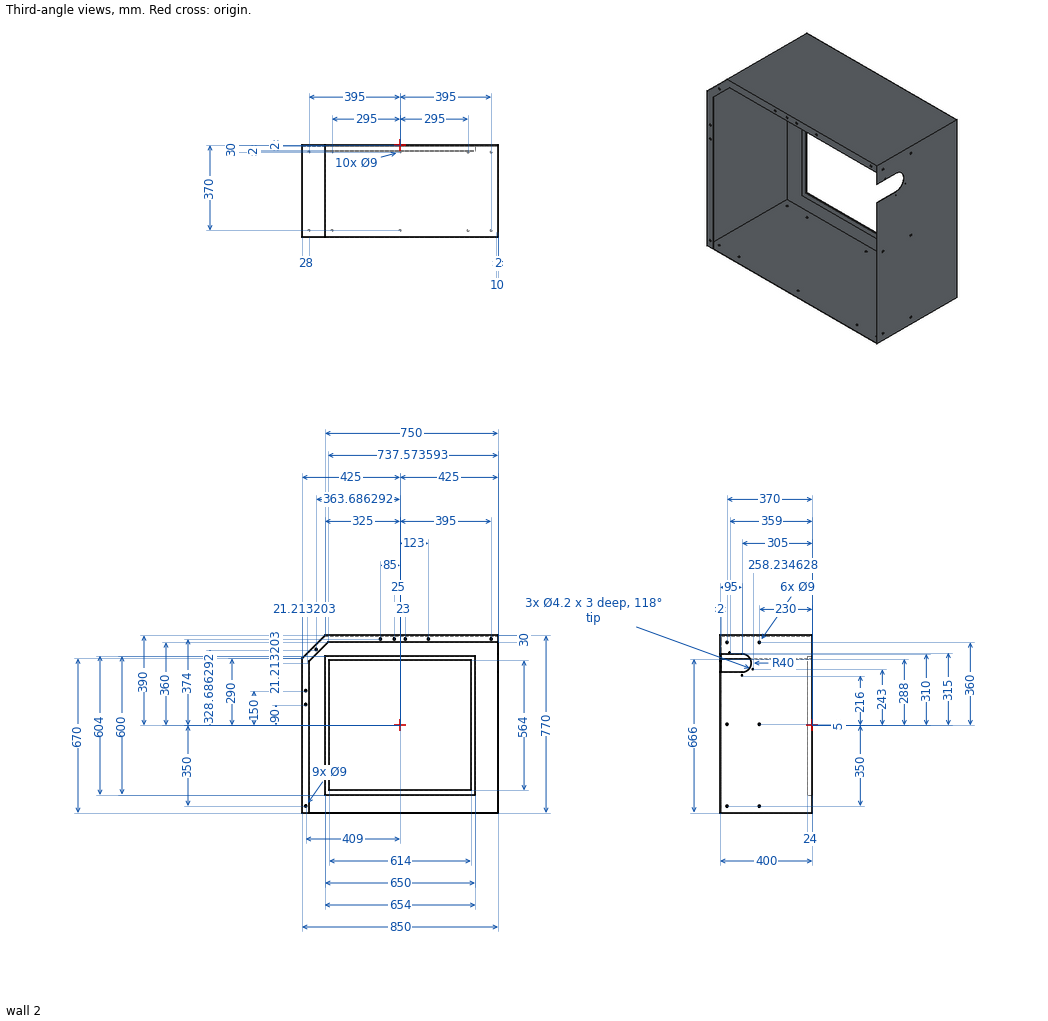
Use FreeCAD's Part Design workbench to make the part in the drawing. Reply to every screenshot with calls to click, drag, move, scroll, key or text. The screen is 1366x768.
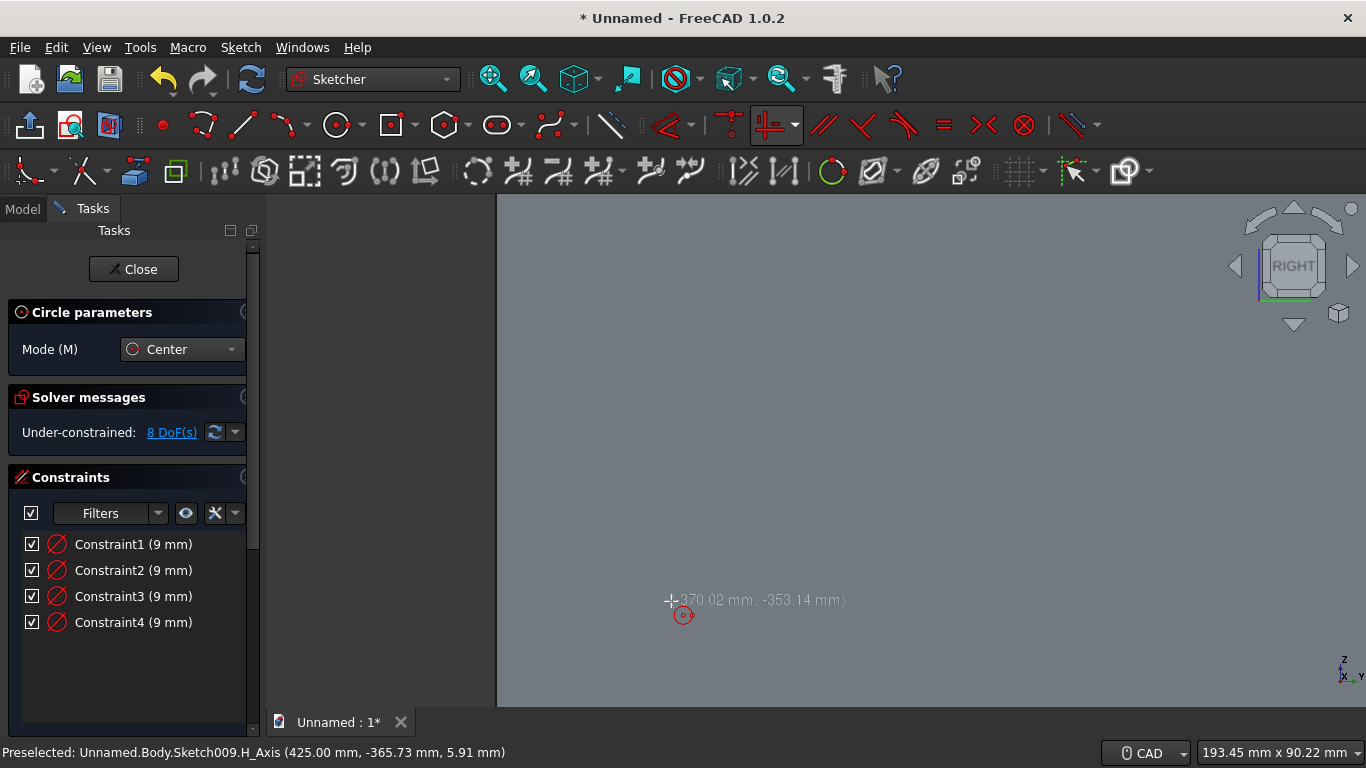
scroll(671, 602, down, 13)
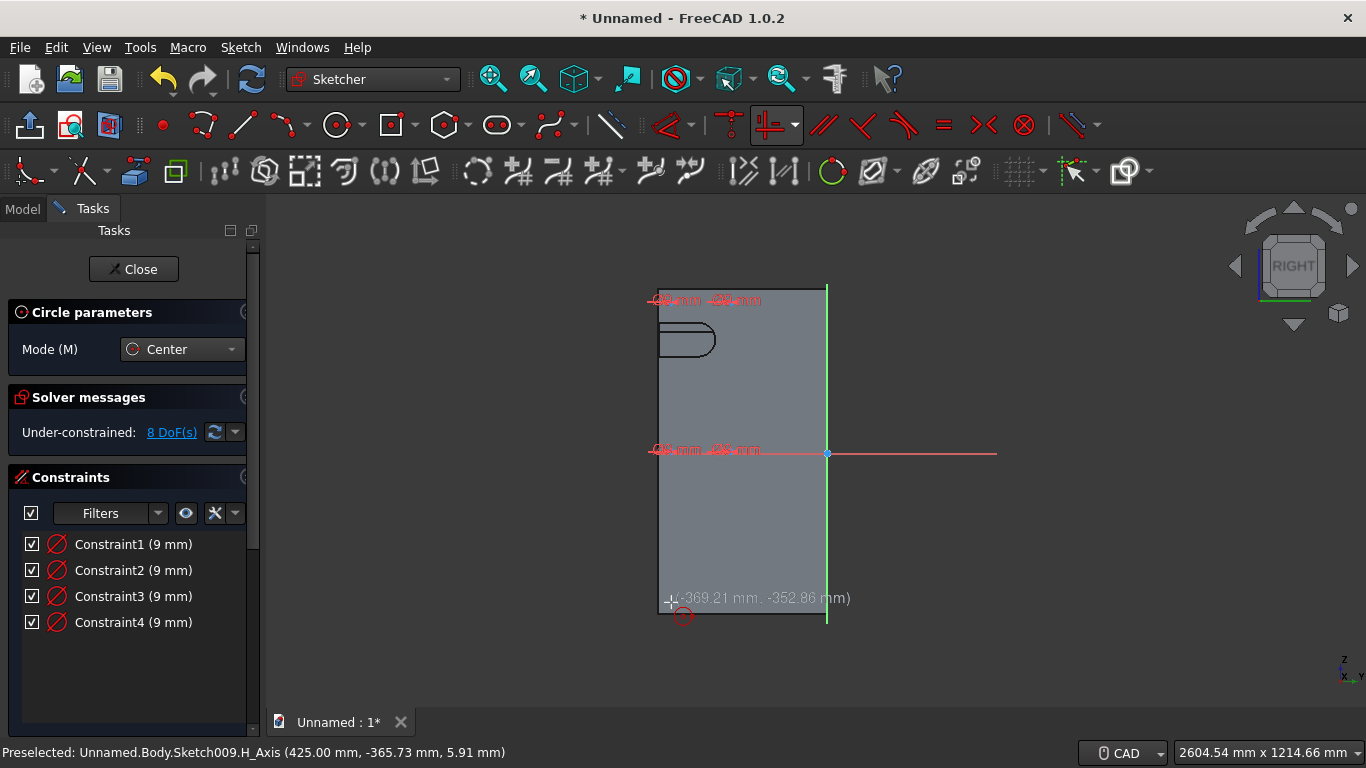
click(671, 602)
move(672, 600)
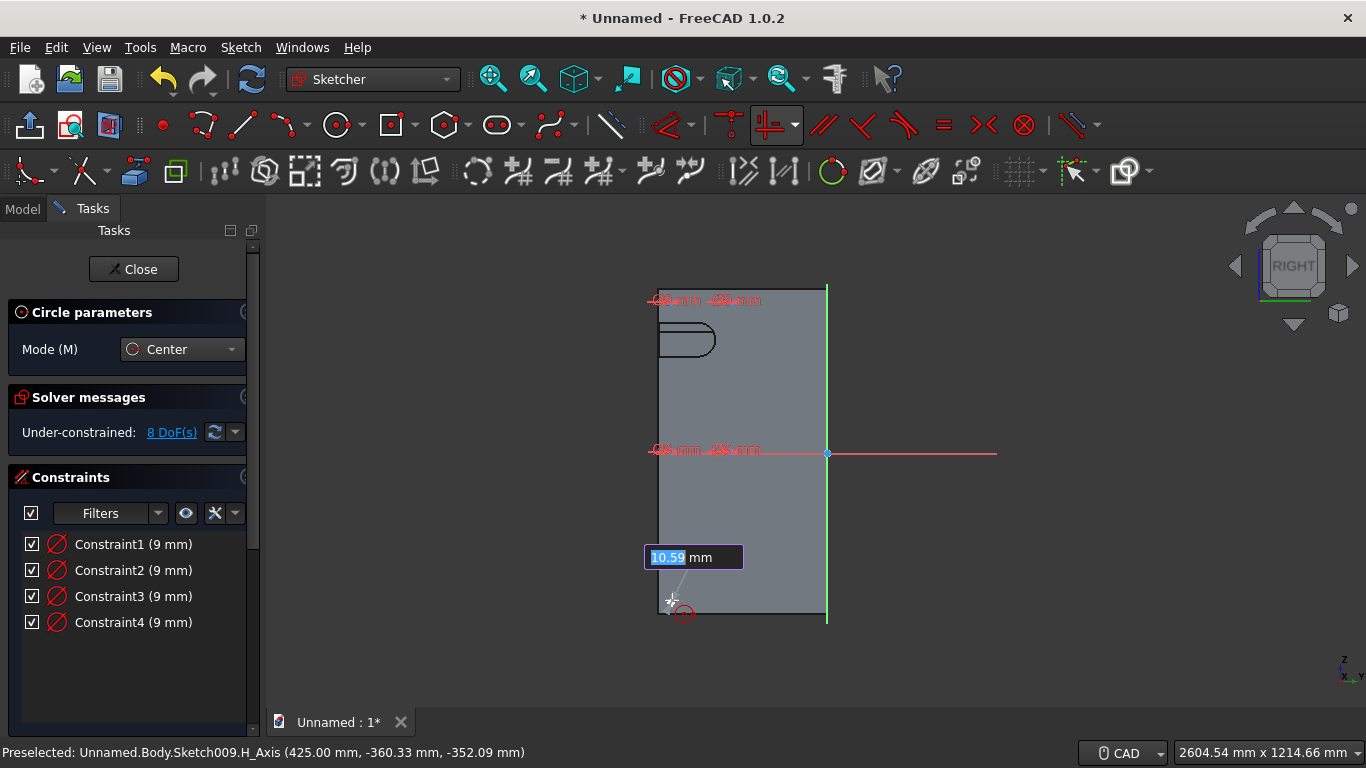
text(9)
key(Return)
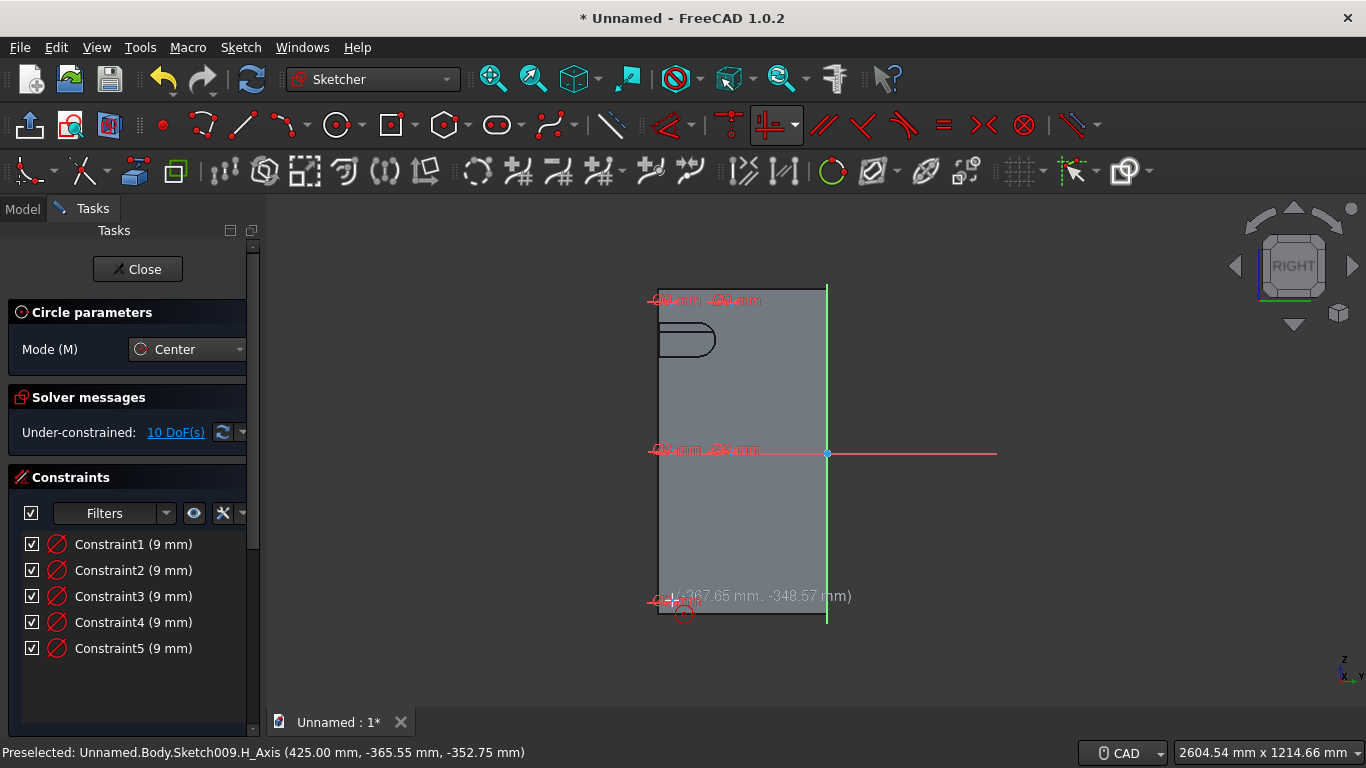
scroll(730, 602, up, 13)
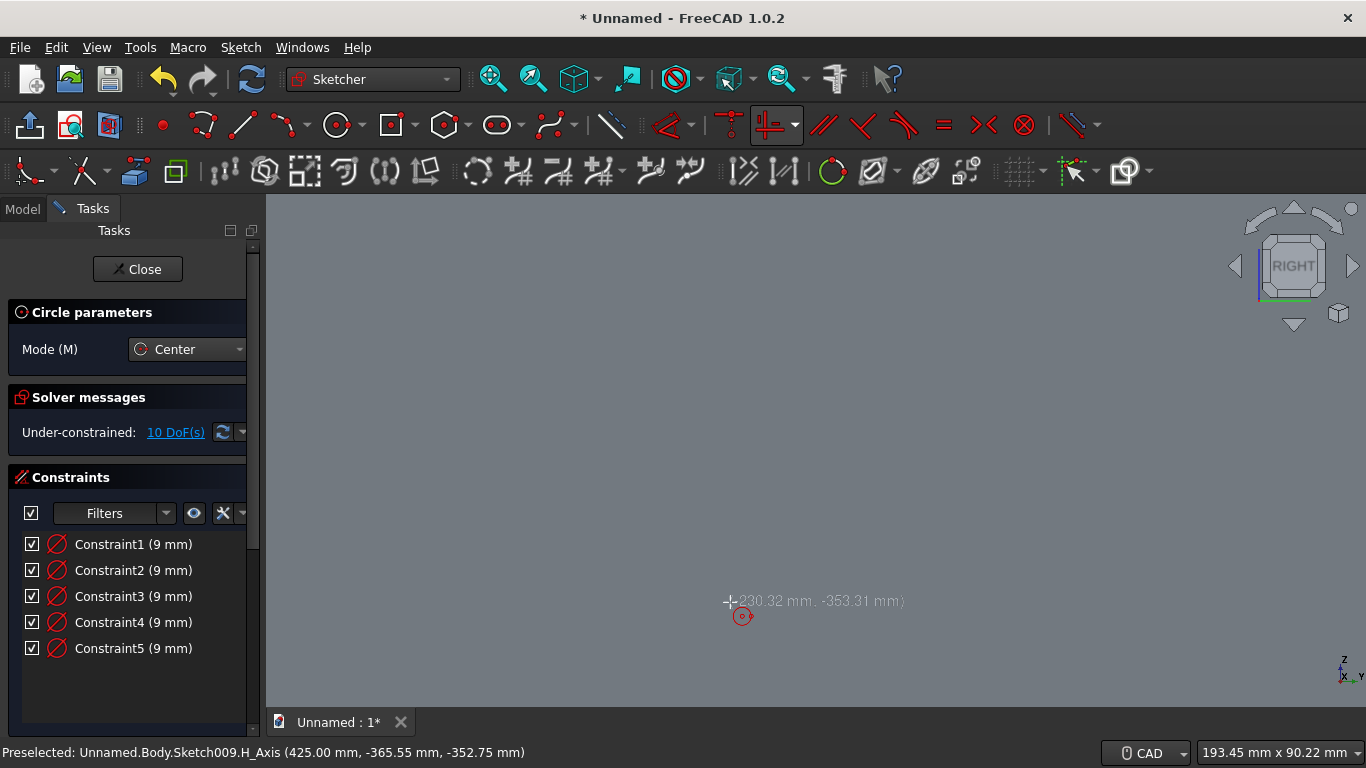
scroll(730, 602, down, 13)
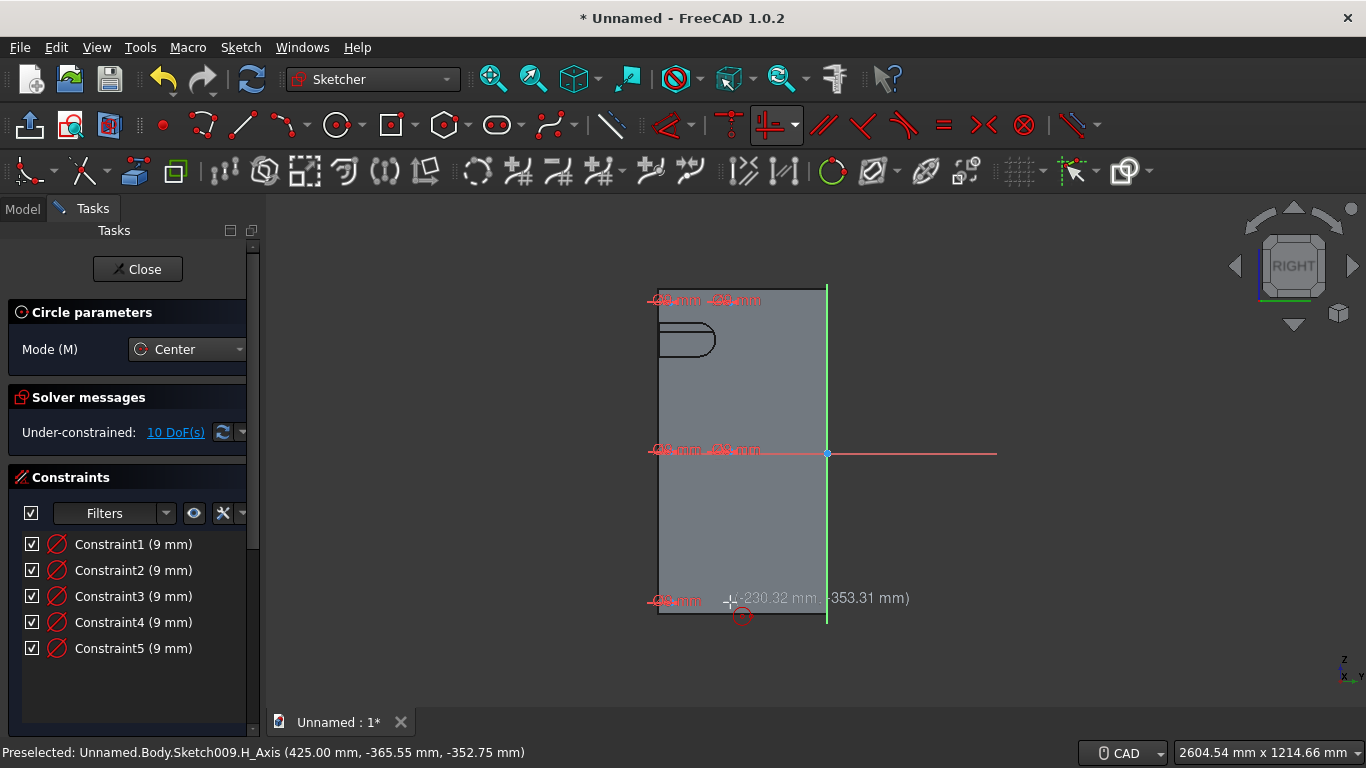
click(730, 602)
move(731, 600)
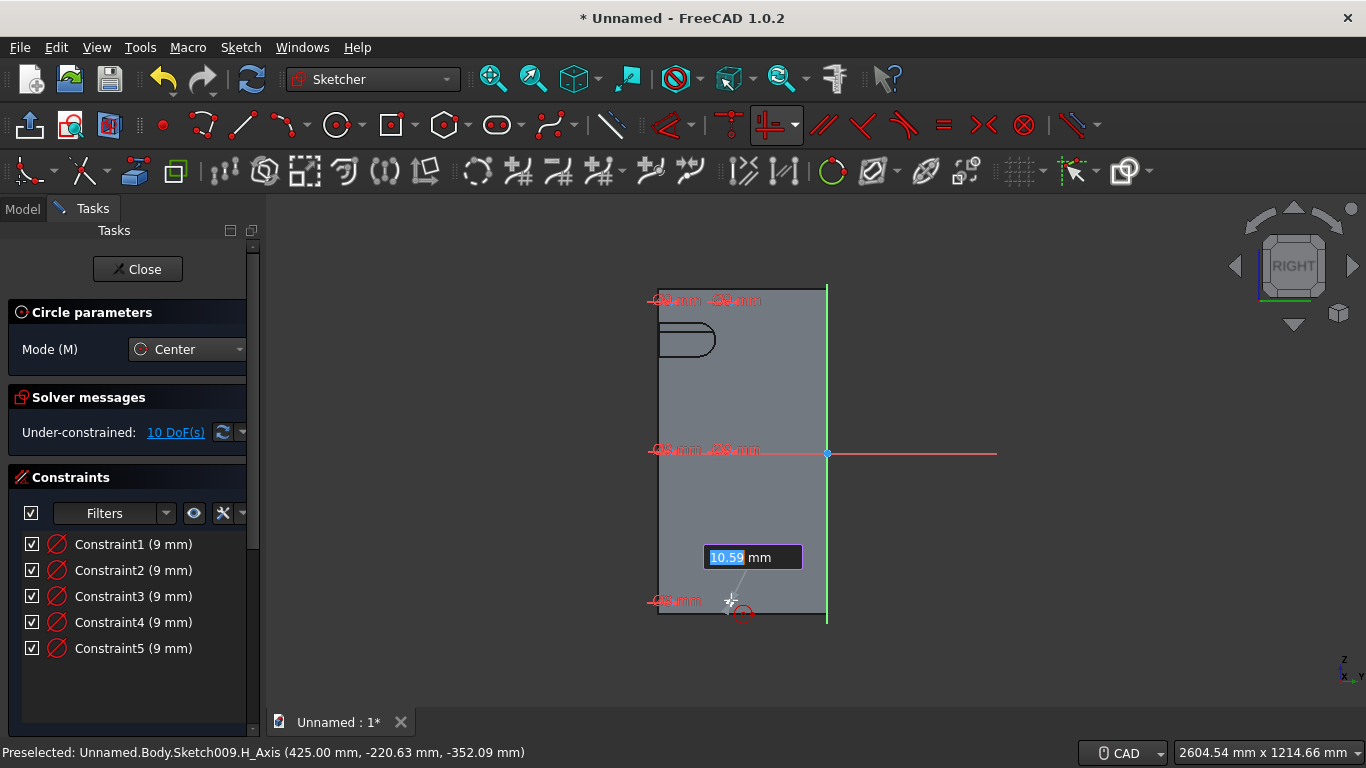
text(9)
key(Return)
key(Escape)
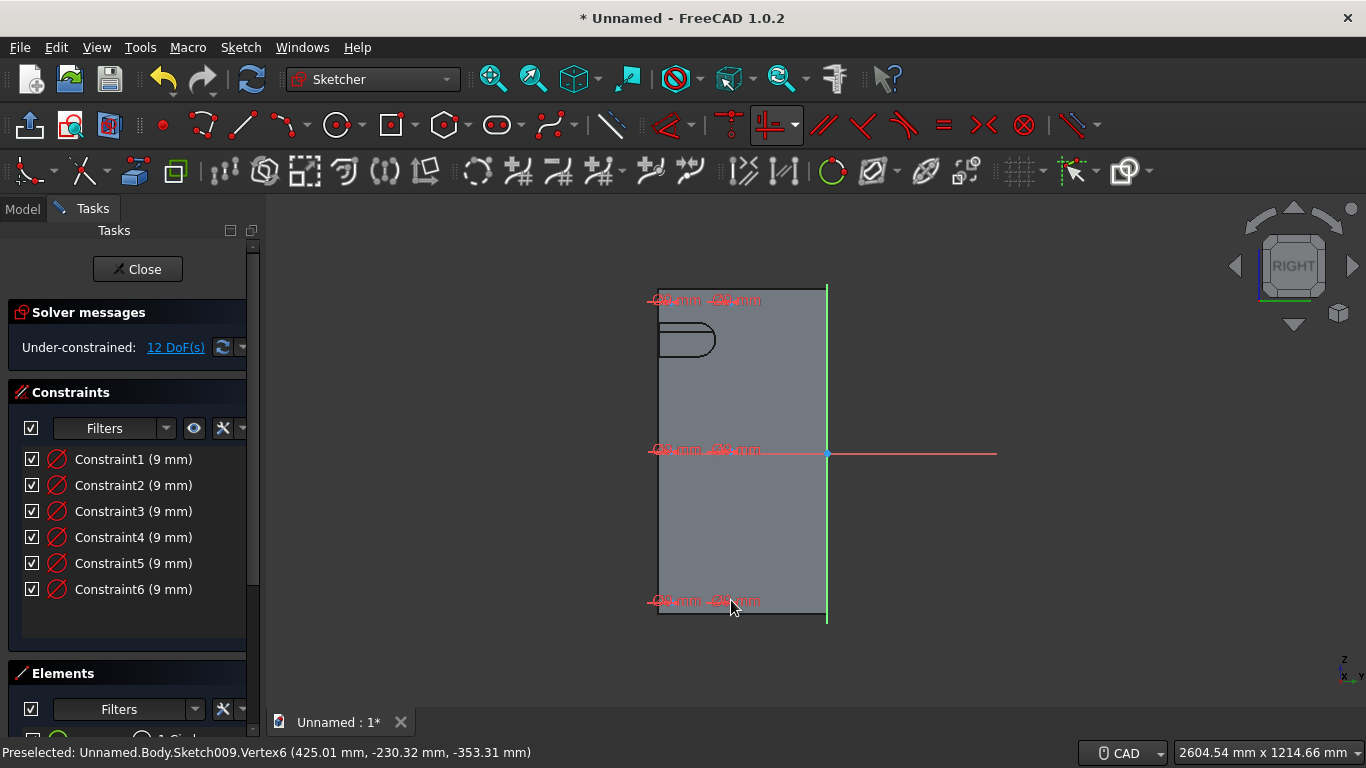
click(731, 302)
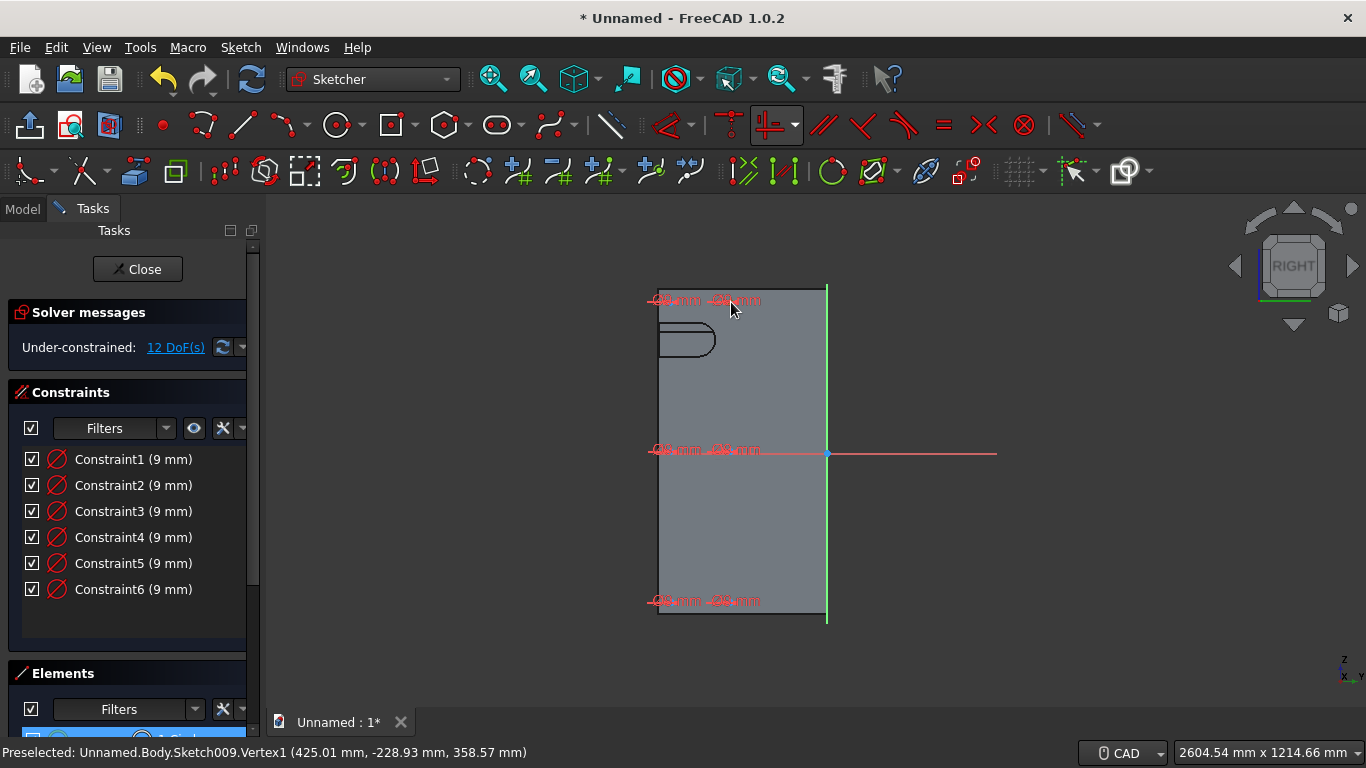
click(671, 302)